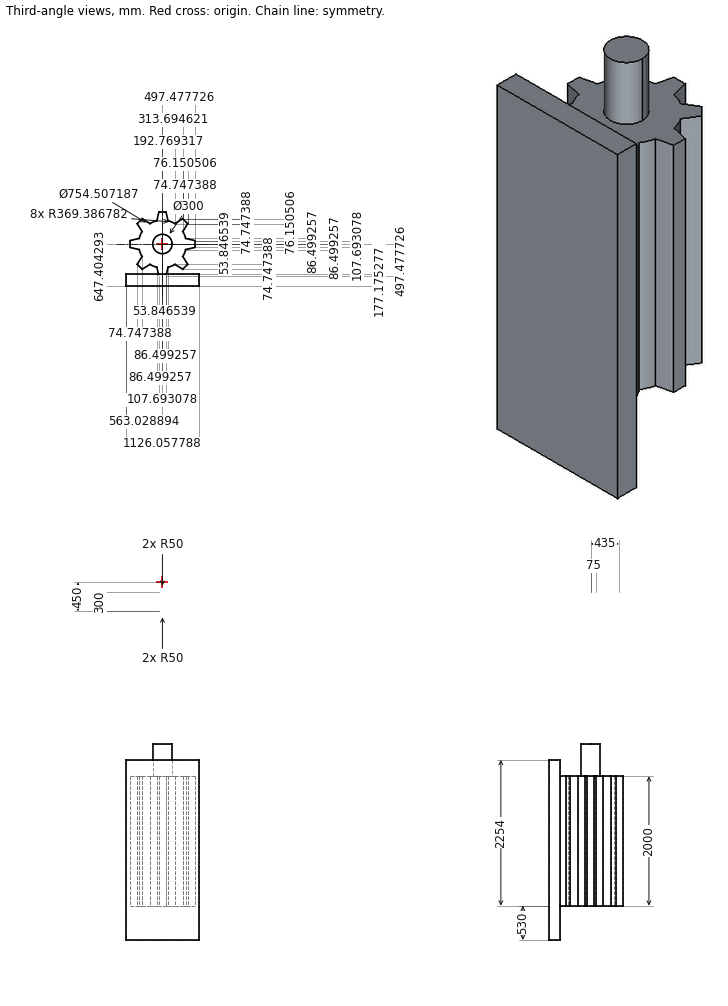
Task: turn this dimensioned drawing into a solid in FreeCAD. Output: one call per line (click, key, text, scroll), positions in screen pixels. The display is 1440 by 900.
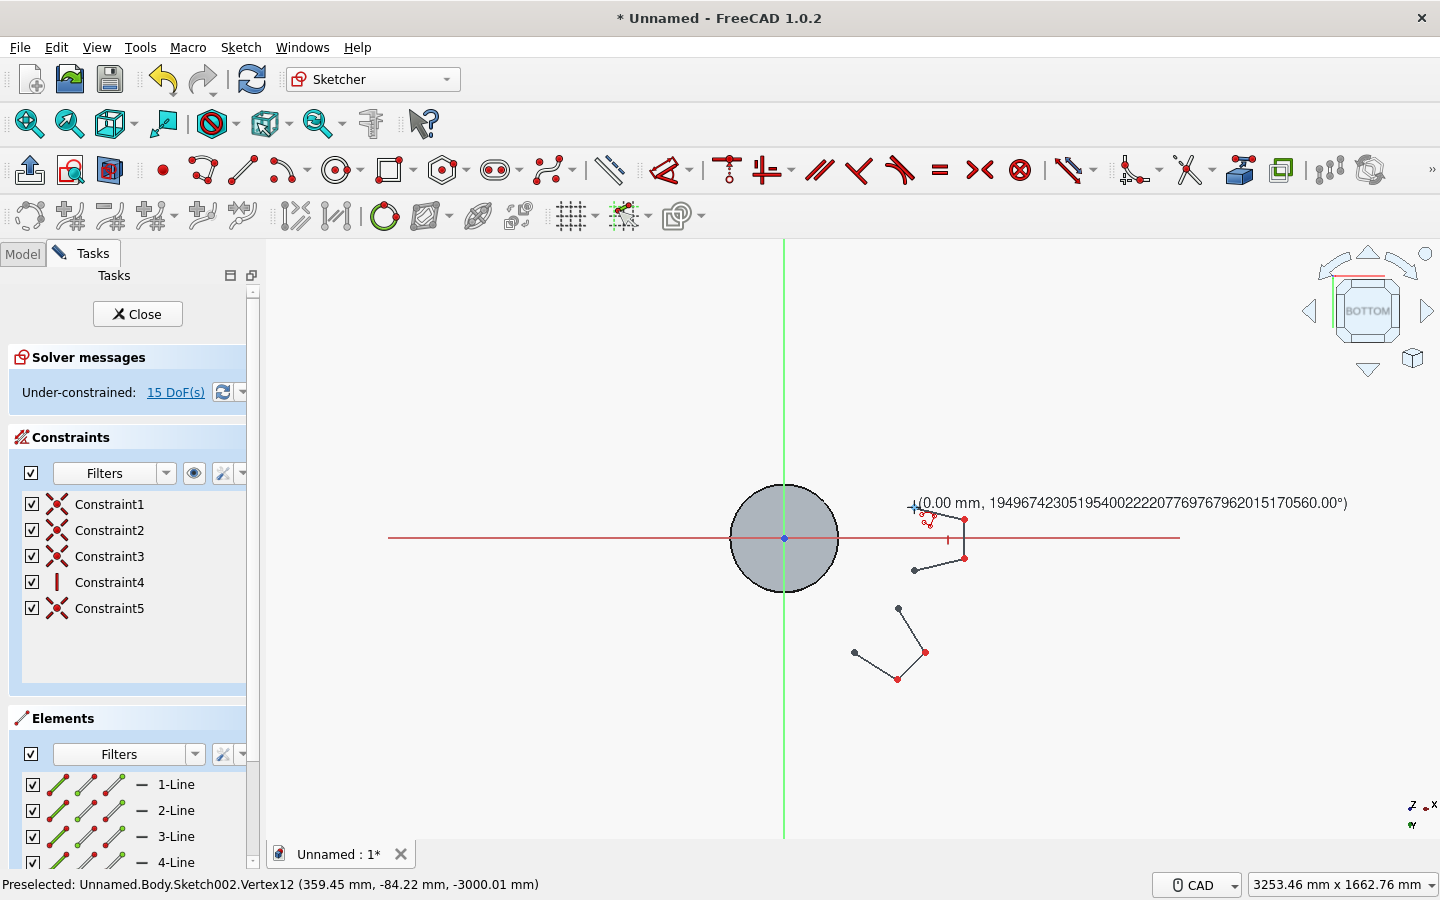
click(898, 469)
click(925, 425)
click(897, 398)
click(854, 425)
right_click(854, 425)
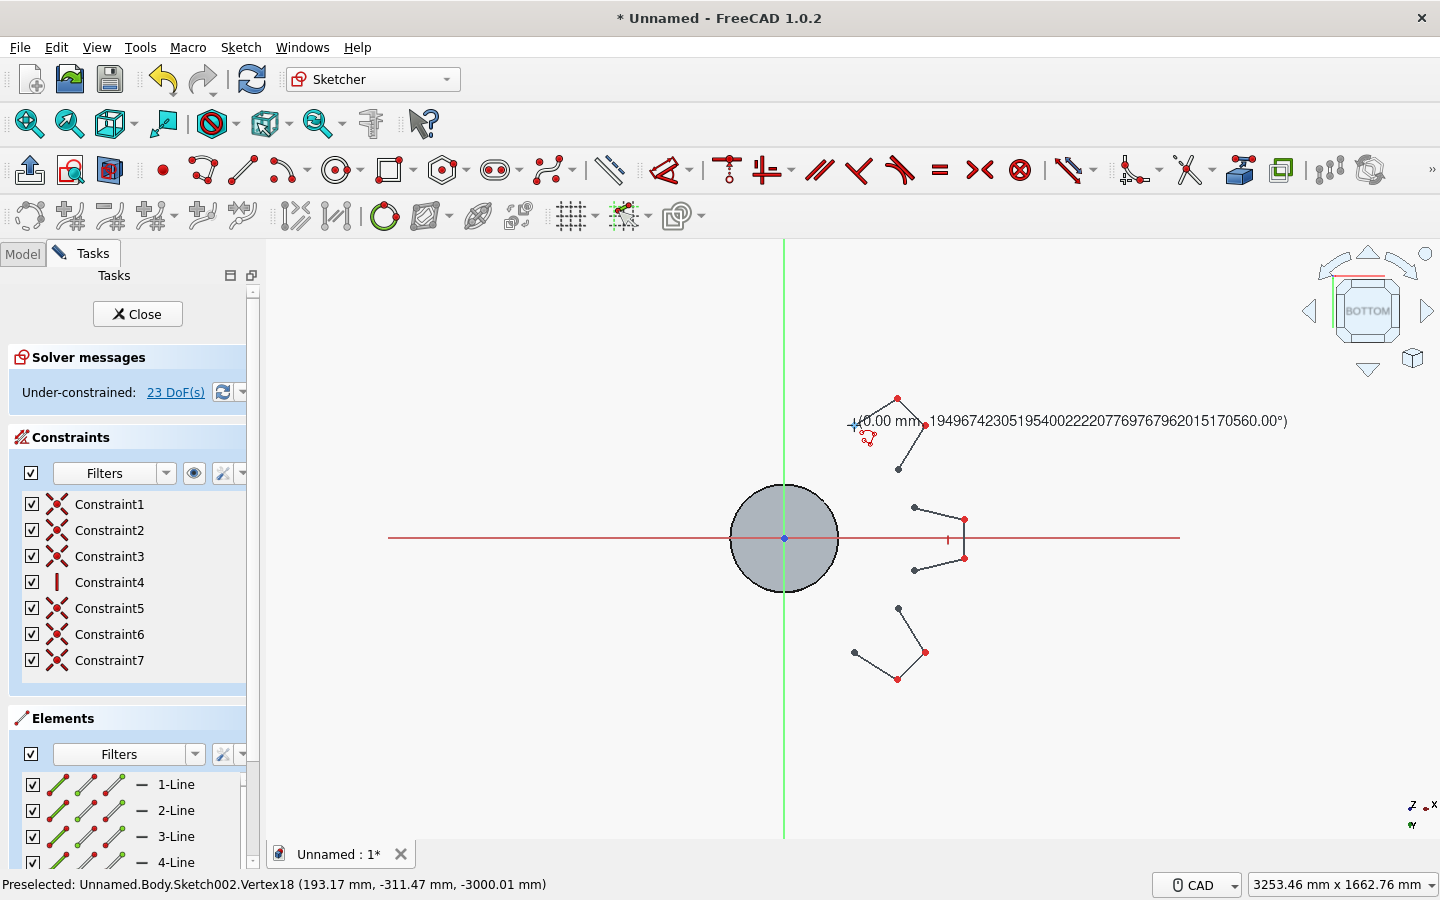
click(816, 409)
click(804, 359)
click(765, 359)
click(753, 409)
right_click(753, 409)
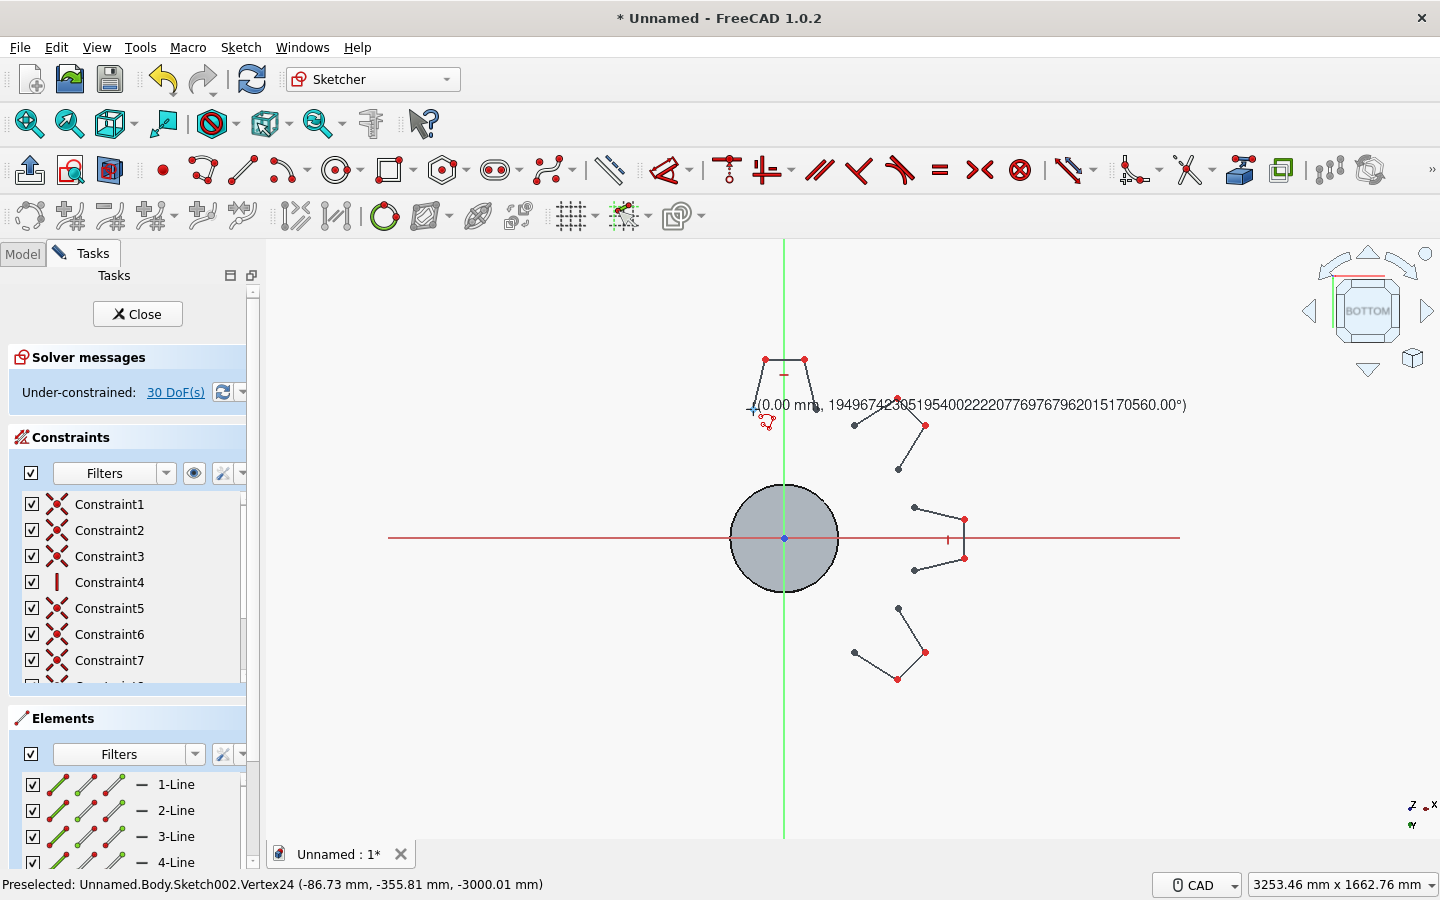
click(715, 425)
click(671, 398)
click(644, 425)
click(671, 469)
right_click(671, 469)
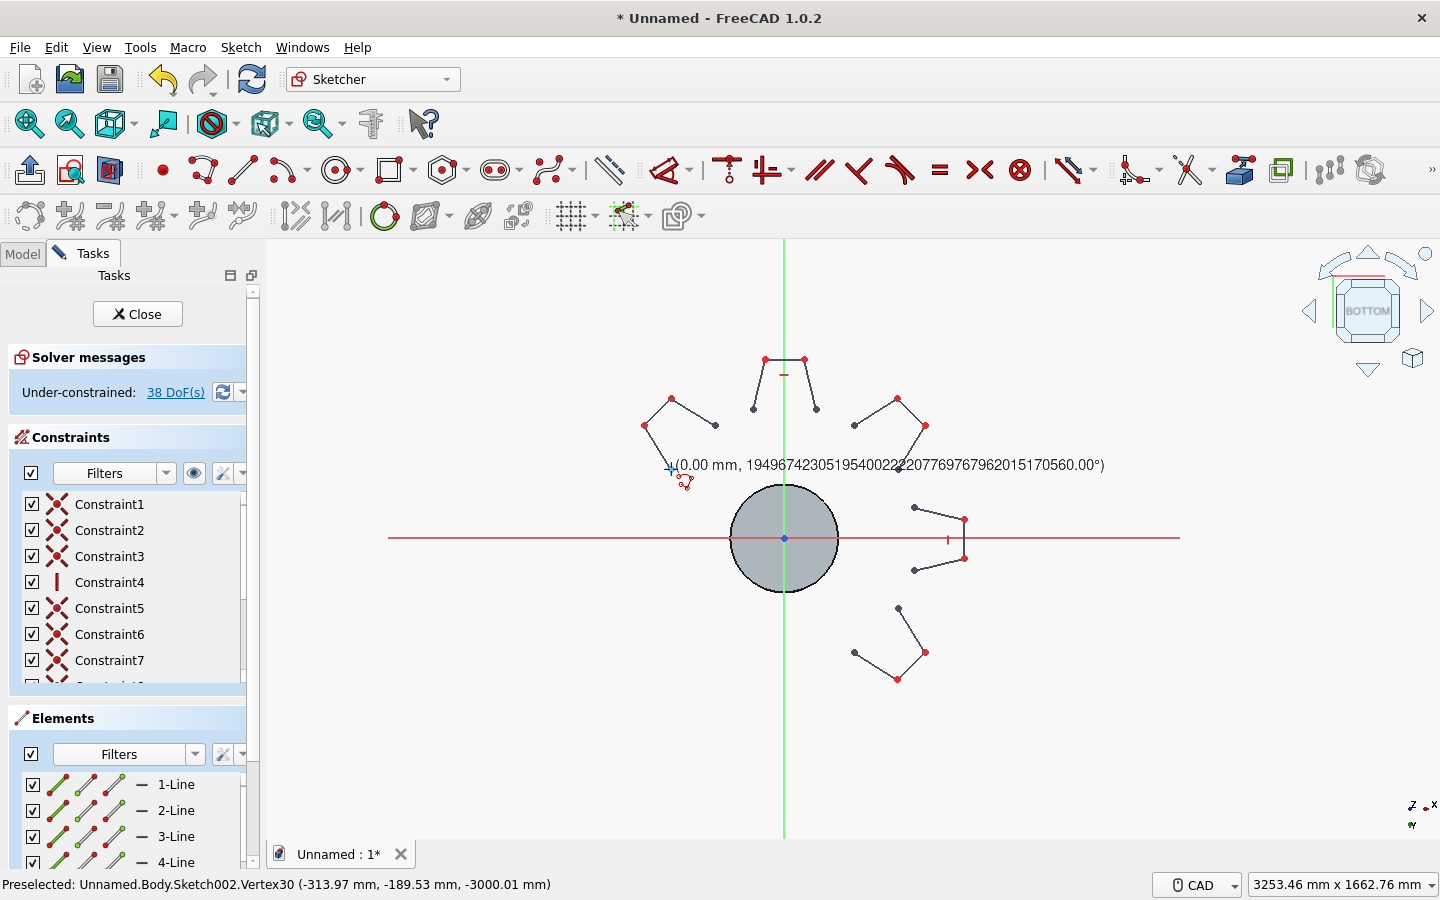
click(655, 507)
click(605, 519)
click(605, 558)
click(655, 570)
right_click(655, 570)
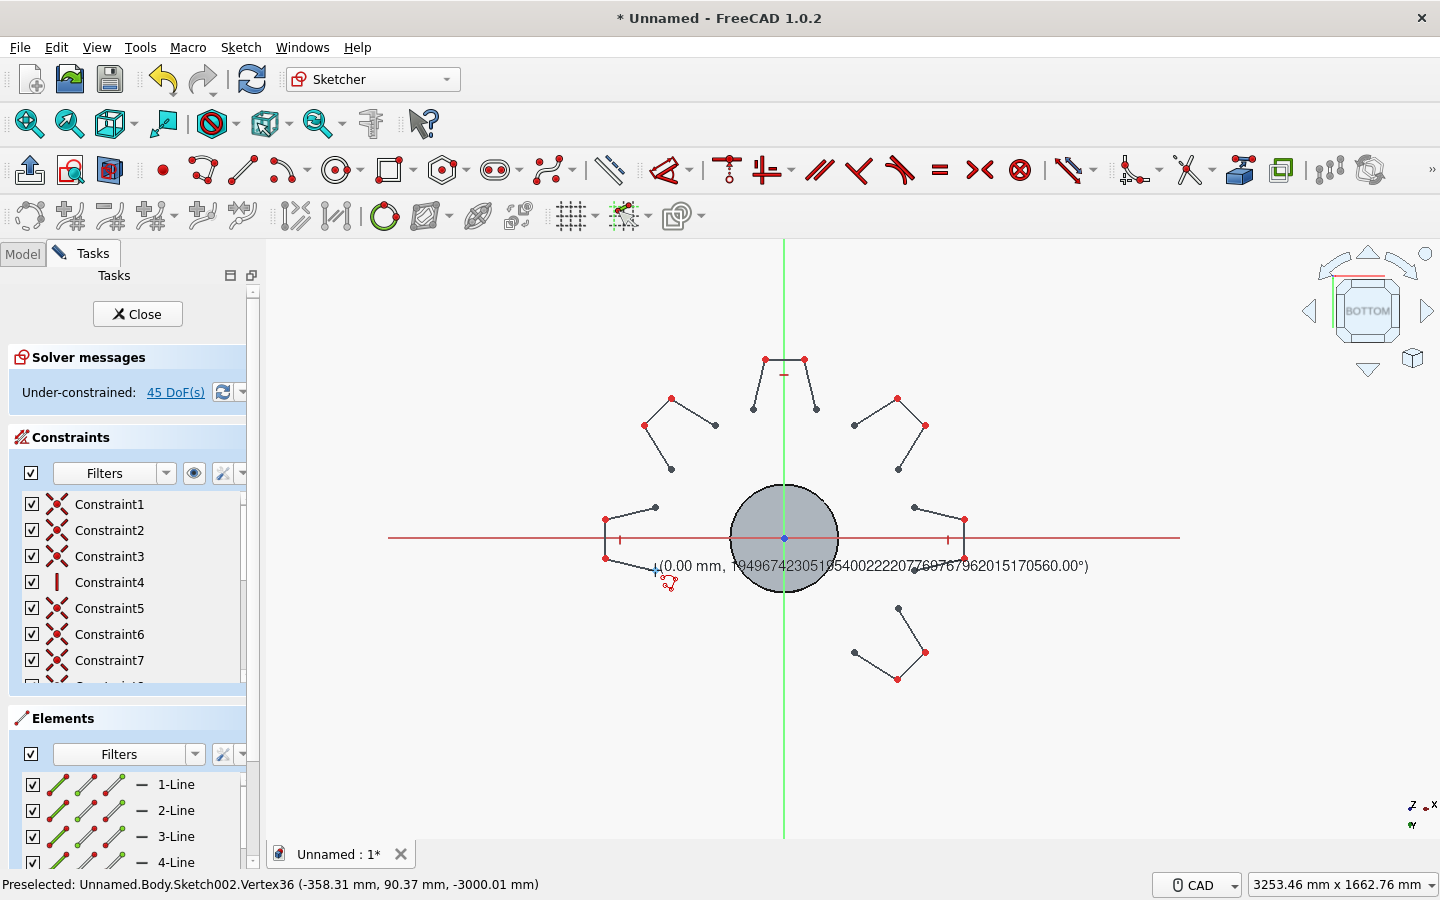
click(671, 608)
click(644, 652)
click(671, 679)
click(715, 652)
right_click(715, 652)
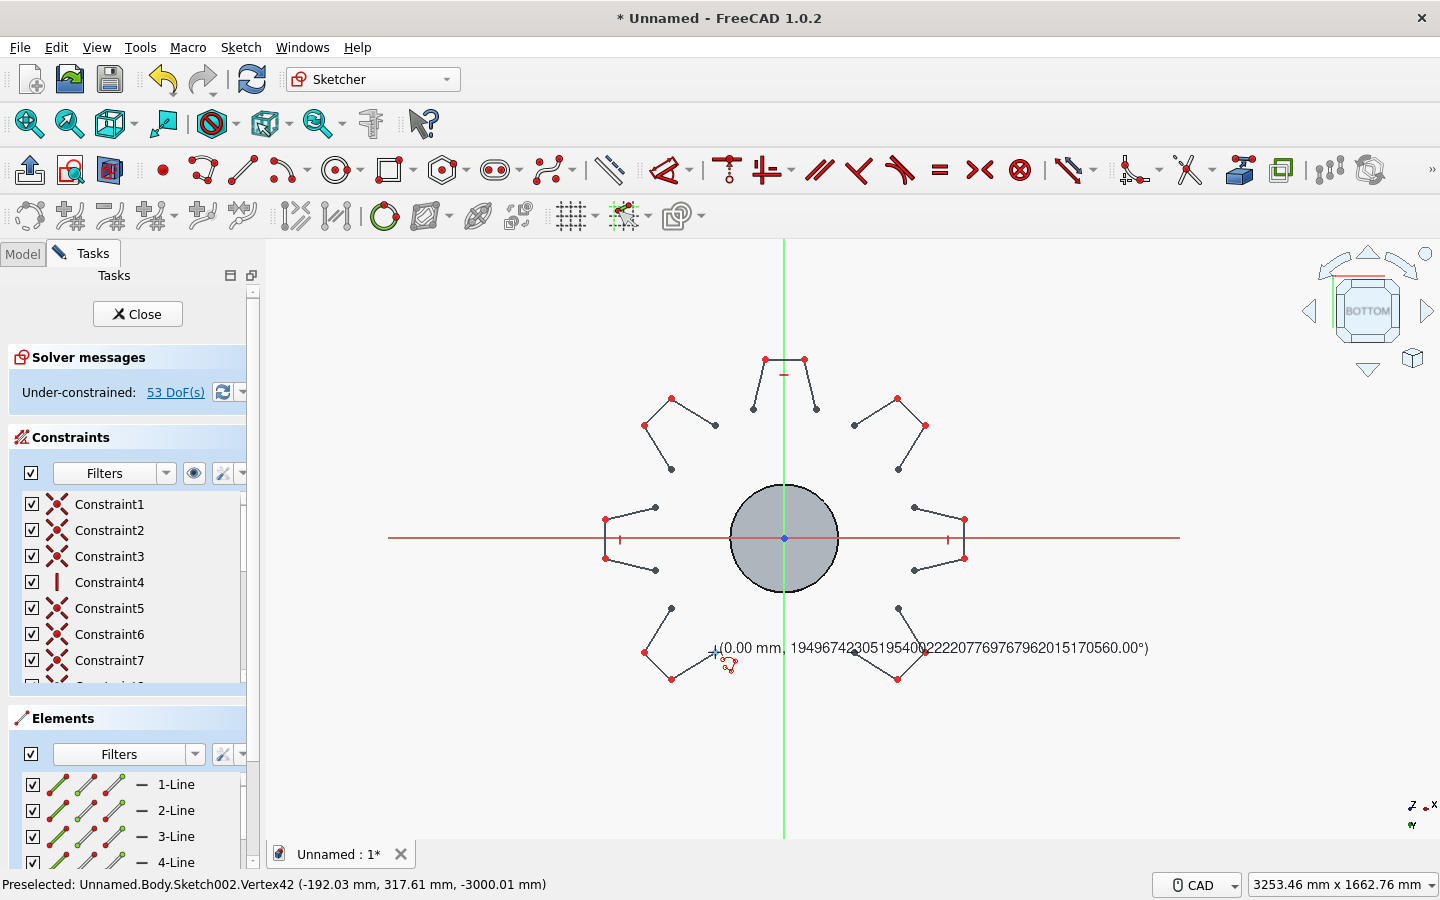
click(753, 668)
click(765, 718)
click(804, 718)
click(816, 668)
right_click(816, 668)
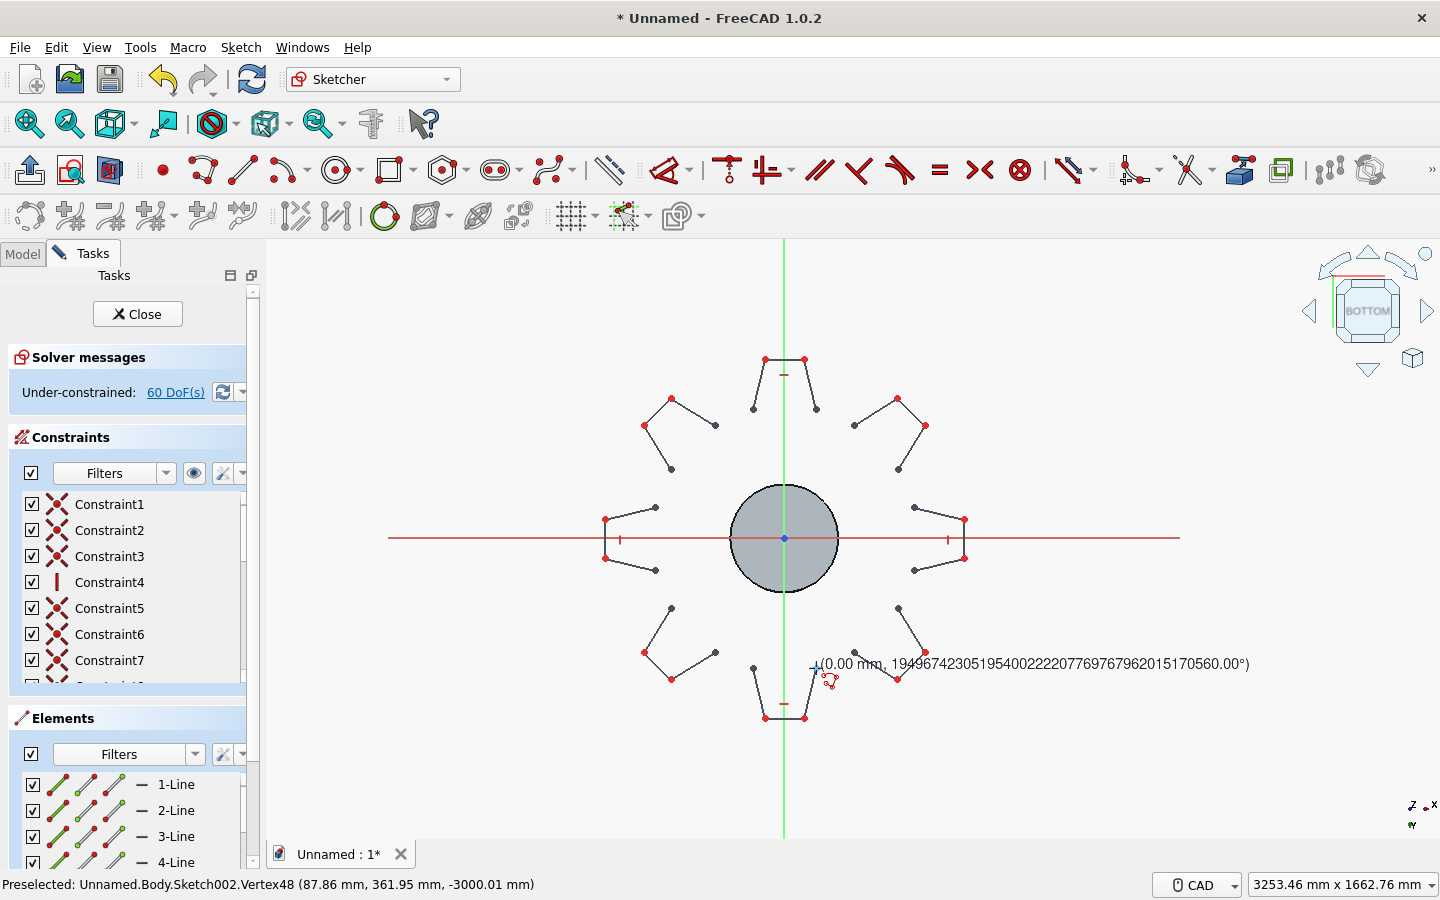
key(g)
key(3)
key(a)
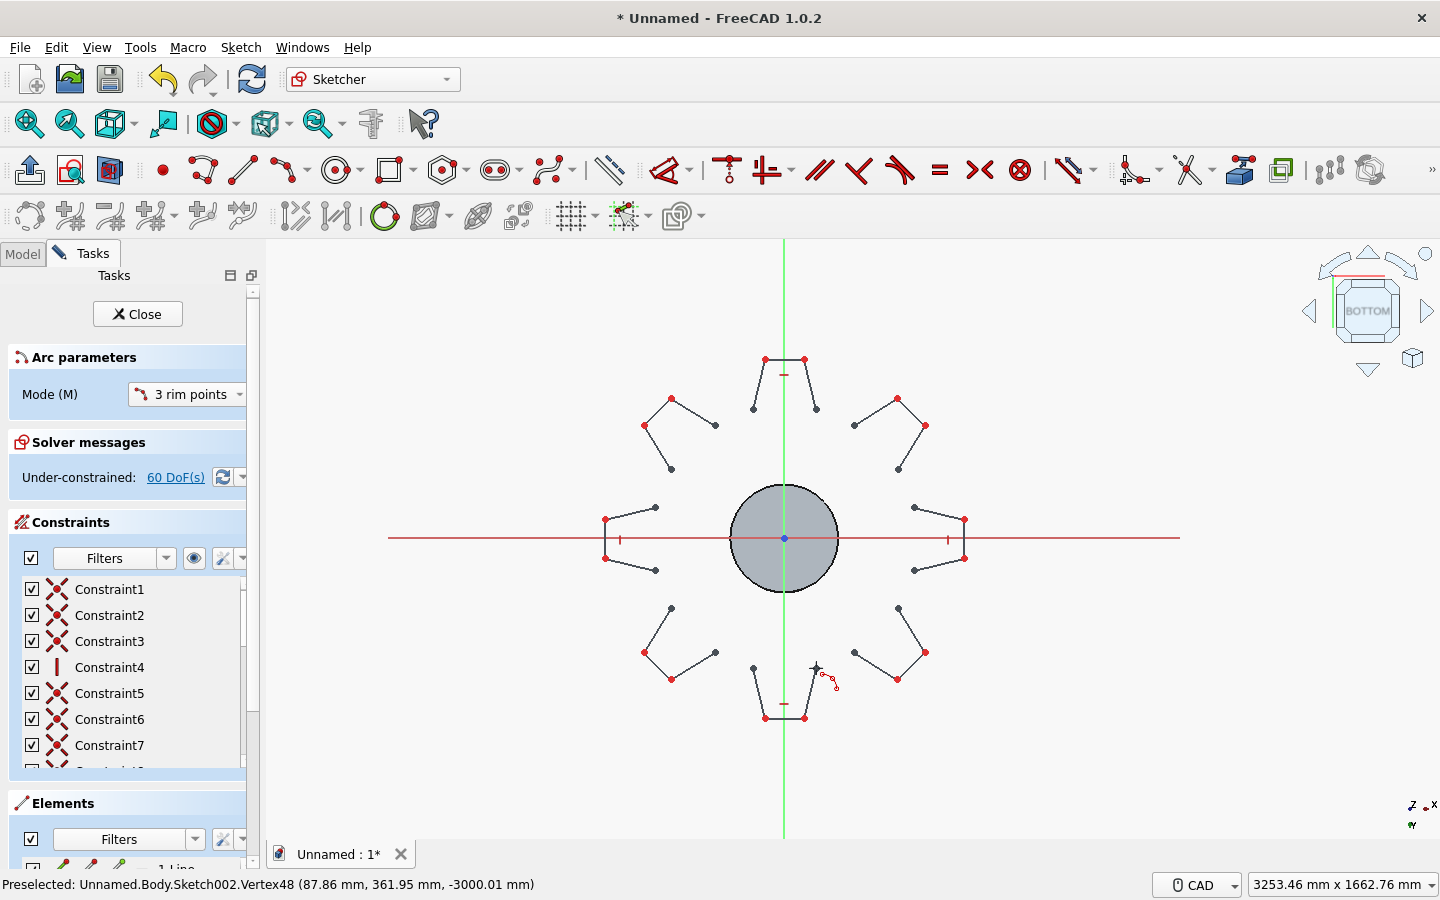
click(898, 609)
click(914, 571)